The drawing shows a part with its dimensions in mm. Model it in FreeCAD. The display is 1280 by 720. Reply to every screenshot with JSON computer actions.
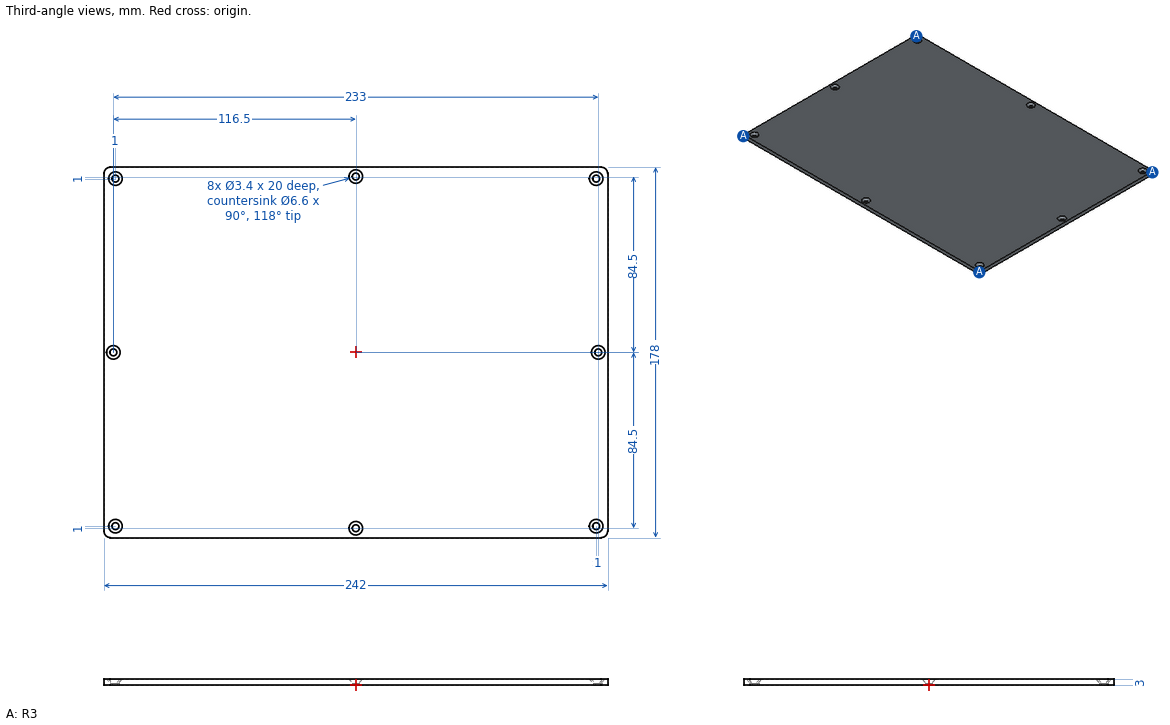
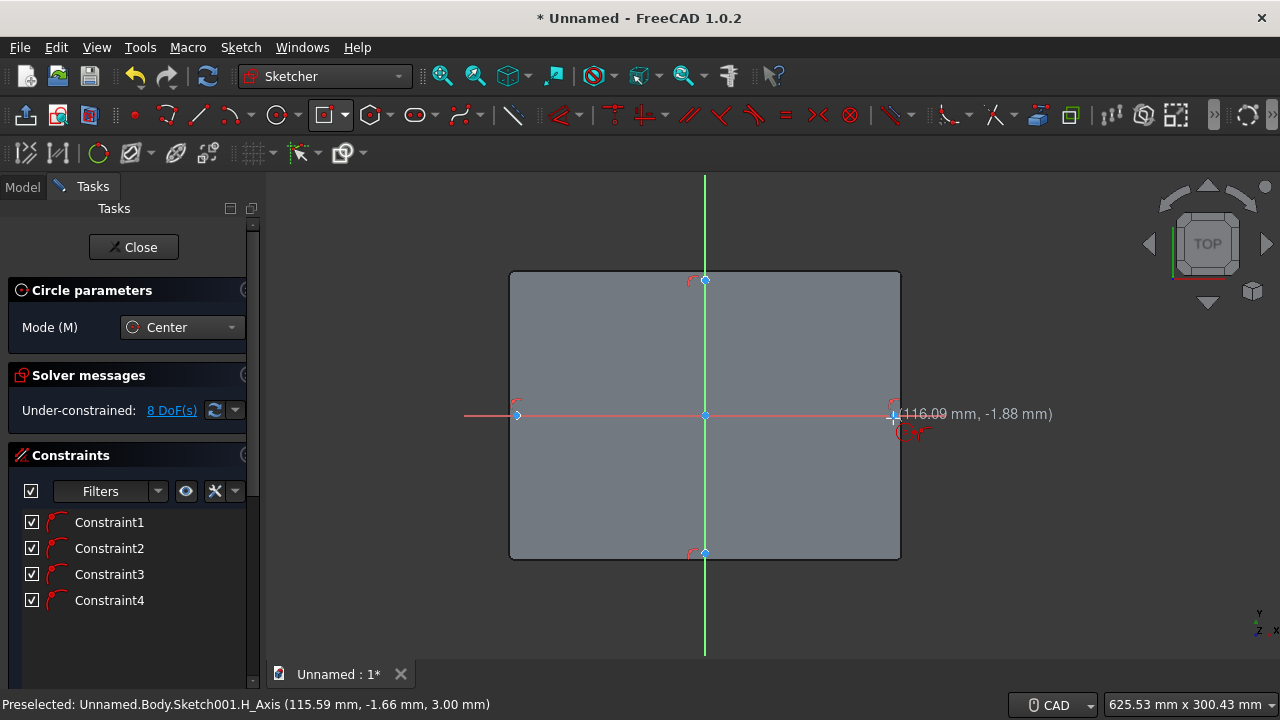
{"action": "scroll", "coordinate": [518, 280], "scroll_direction": "up", "scroll_amount": 11}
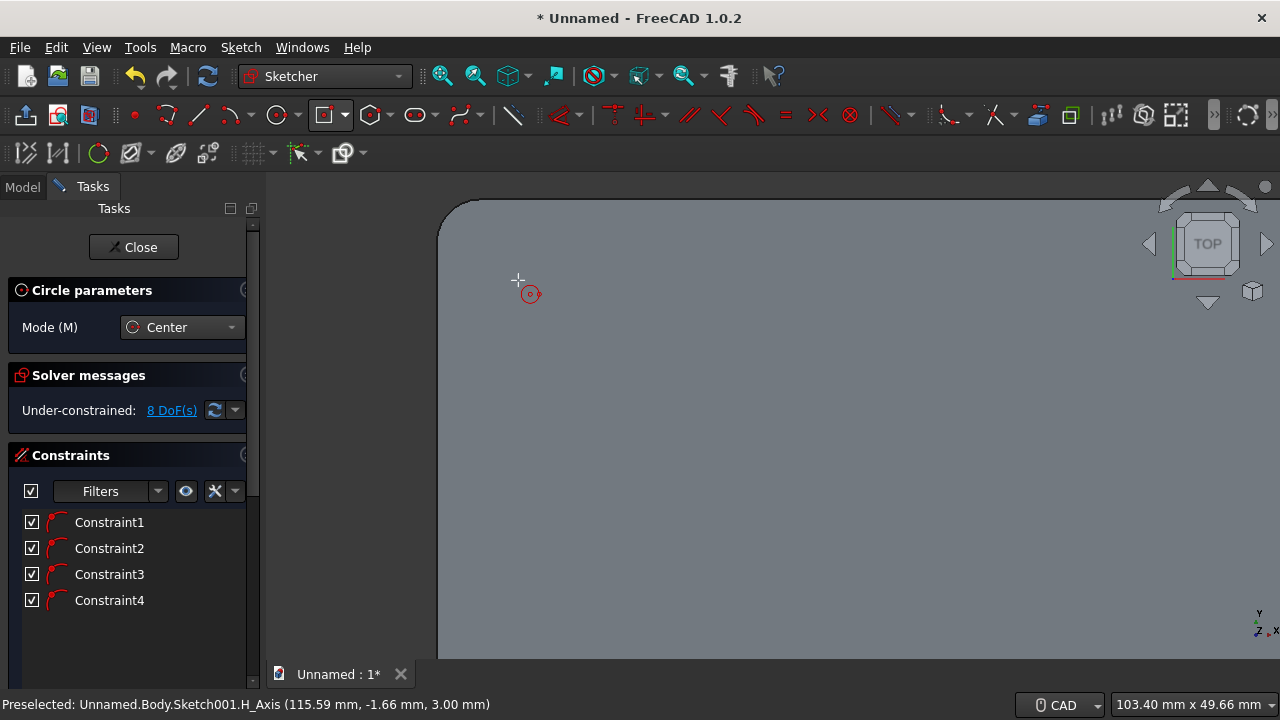
{"action": "scroll", "coordinate": [517, 280], "scroll_direction": "down", "scroll_amount": 11}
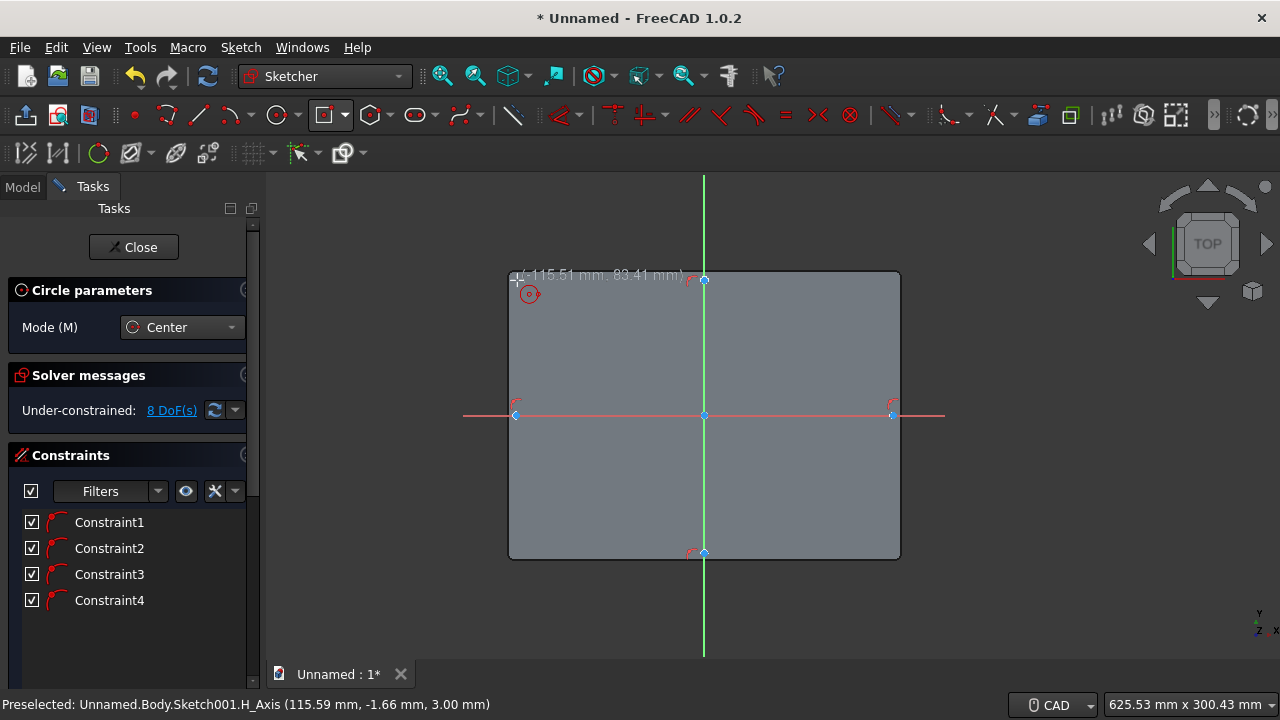
{"action": "left_click", "coordinate": [517, 280]}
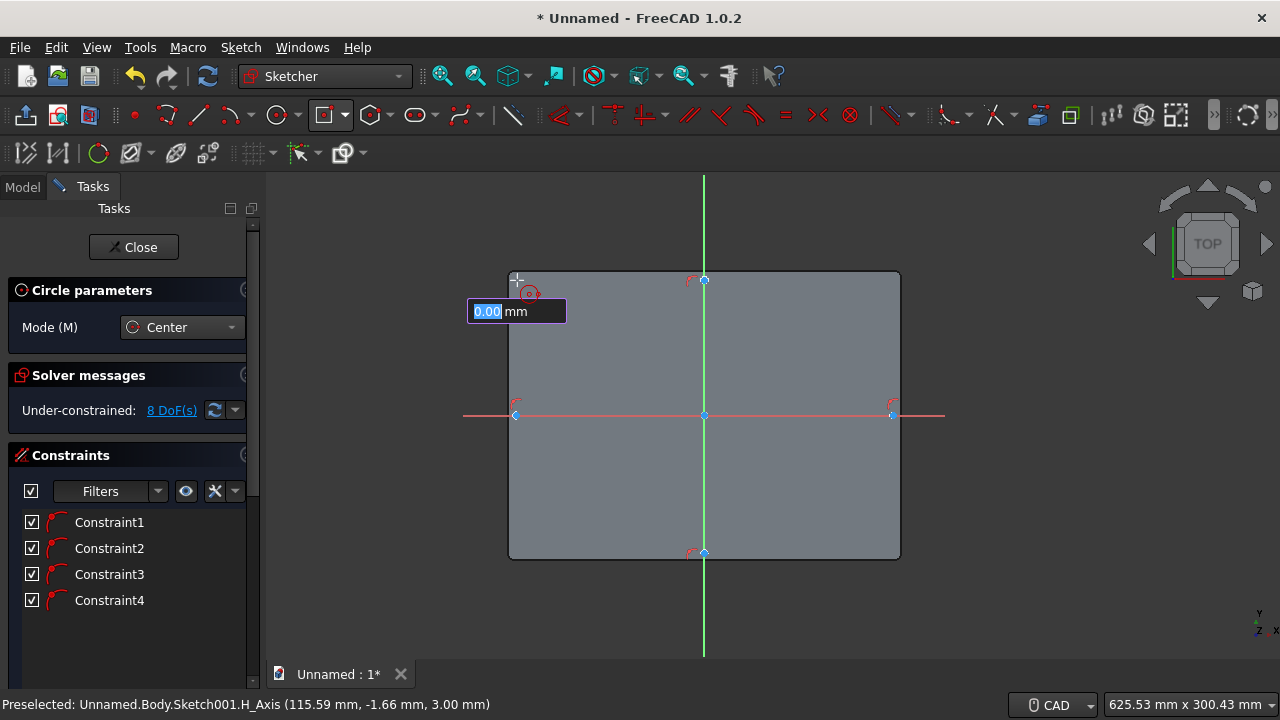
{"action": "scroll", "coordinate": [519, 278], "scroll_direction": "up", "scroll_amount": 9}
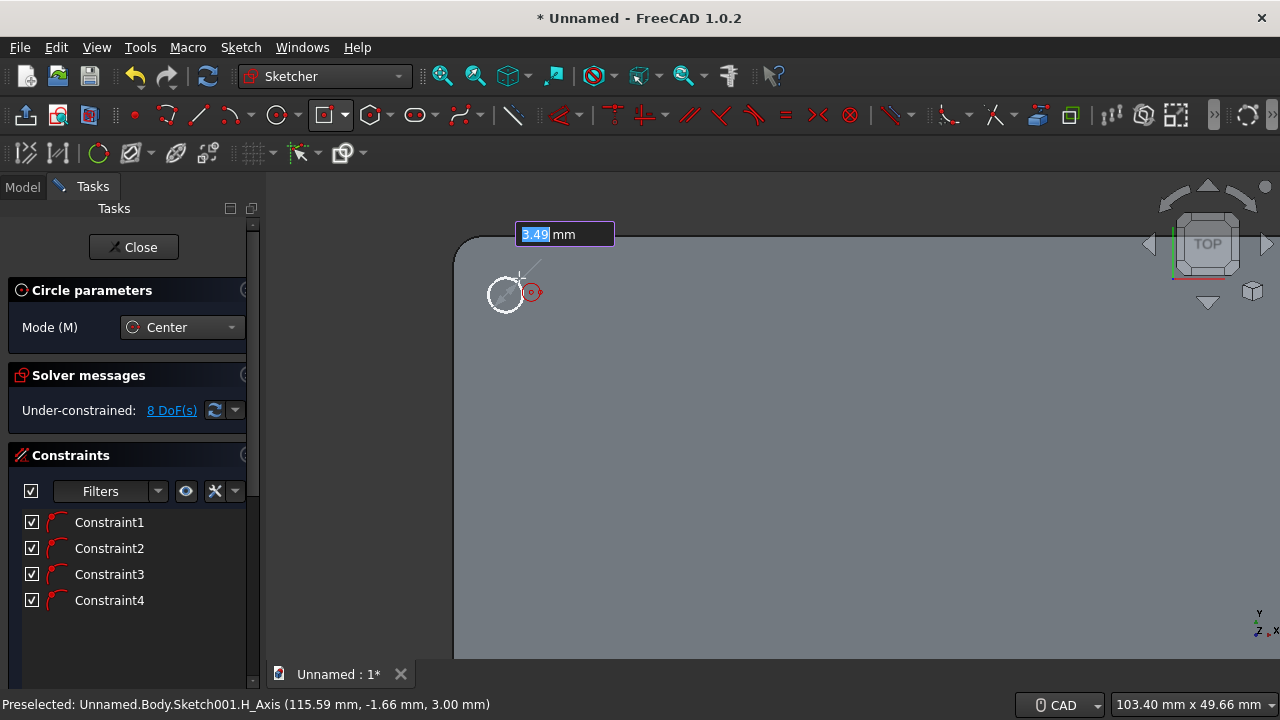
{"action": "left_click", "coordinate": [519, 278]}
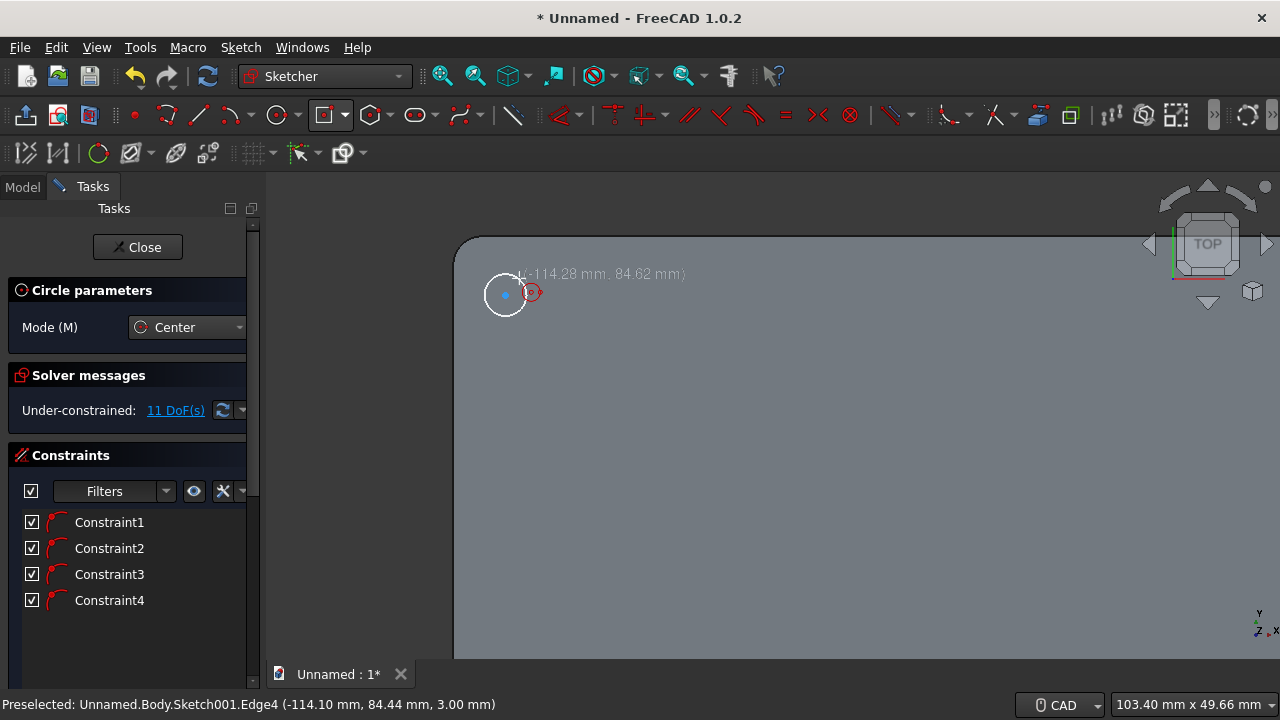
{"action": "scroll", "coordinate": [519, 278], "scroll_direction": "down", "scroll_amount": 9}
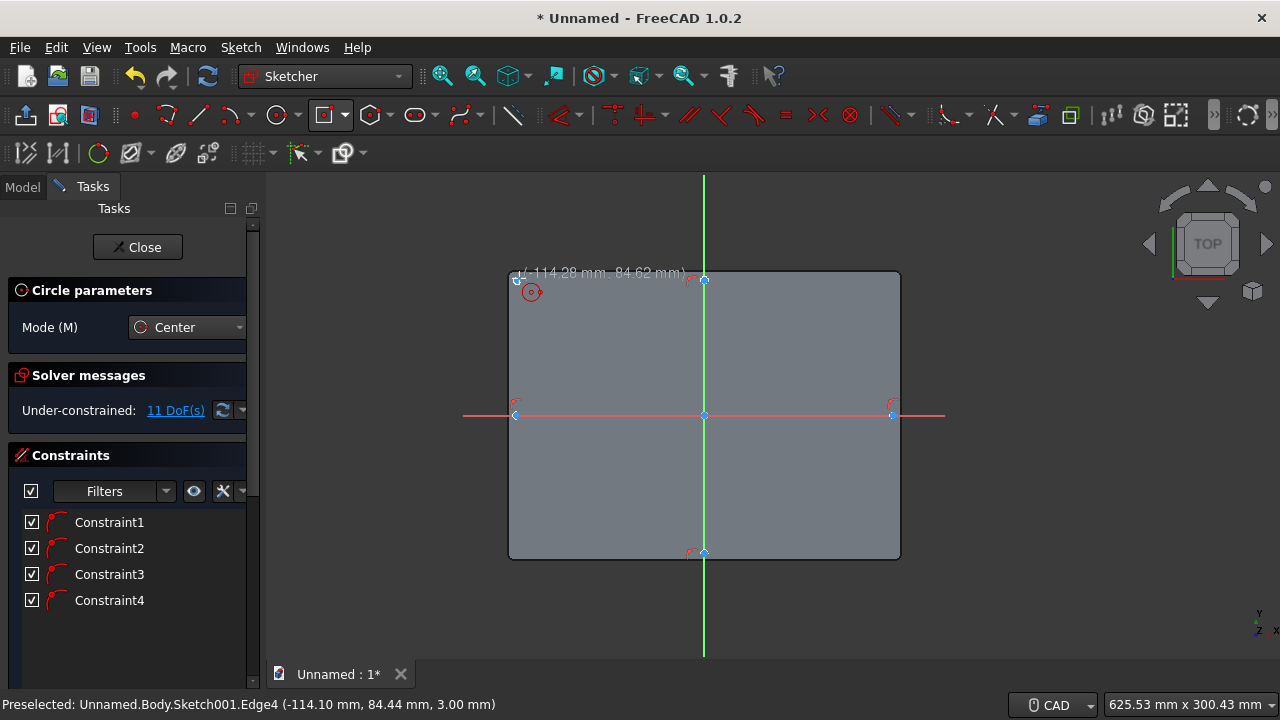
{"action": "scroll", "coordinate": [517, 551], "scroll_direction": "up", "scroll_amount": 11}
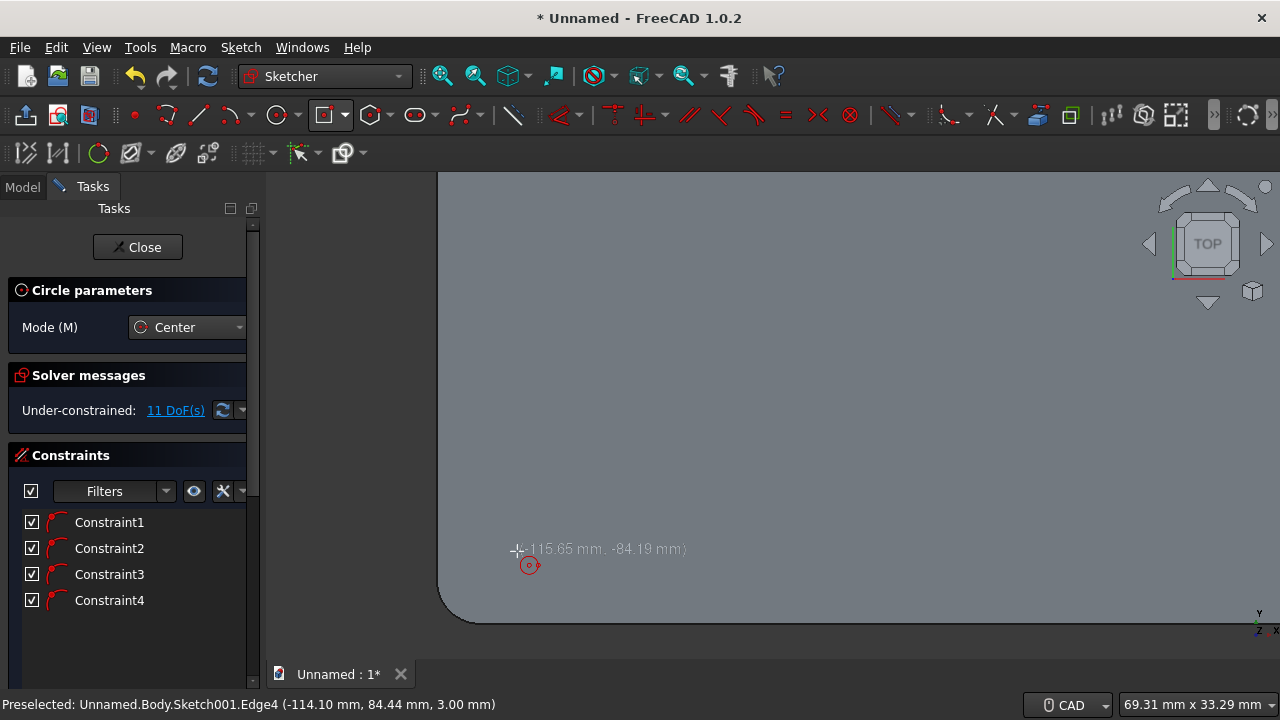
{"action": "scroll", "coordinate": [517, 552], "scroll_direction": "down", "scroll_amount": 11}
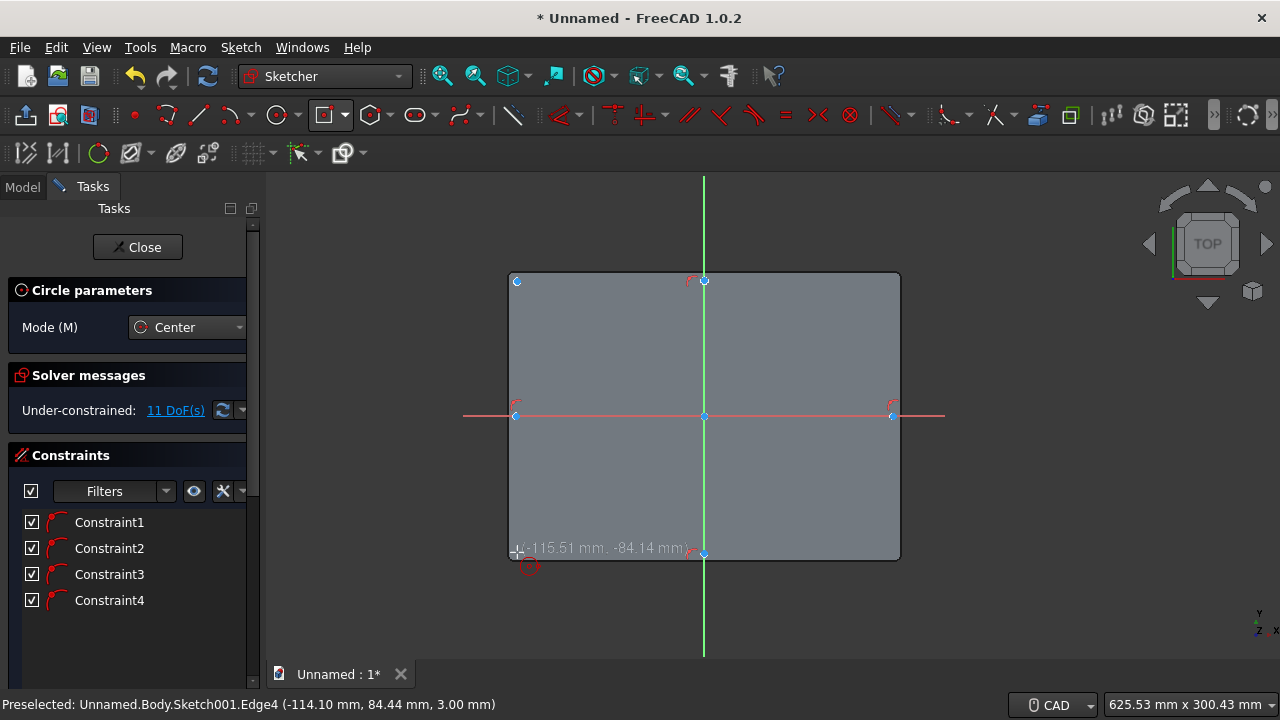
{"action": "left_click", "coordinate": [517, 552]}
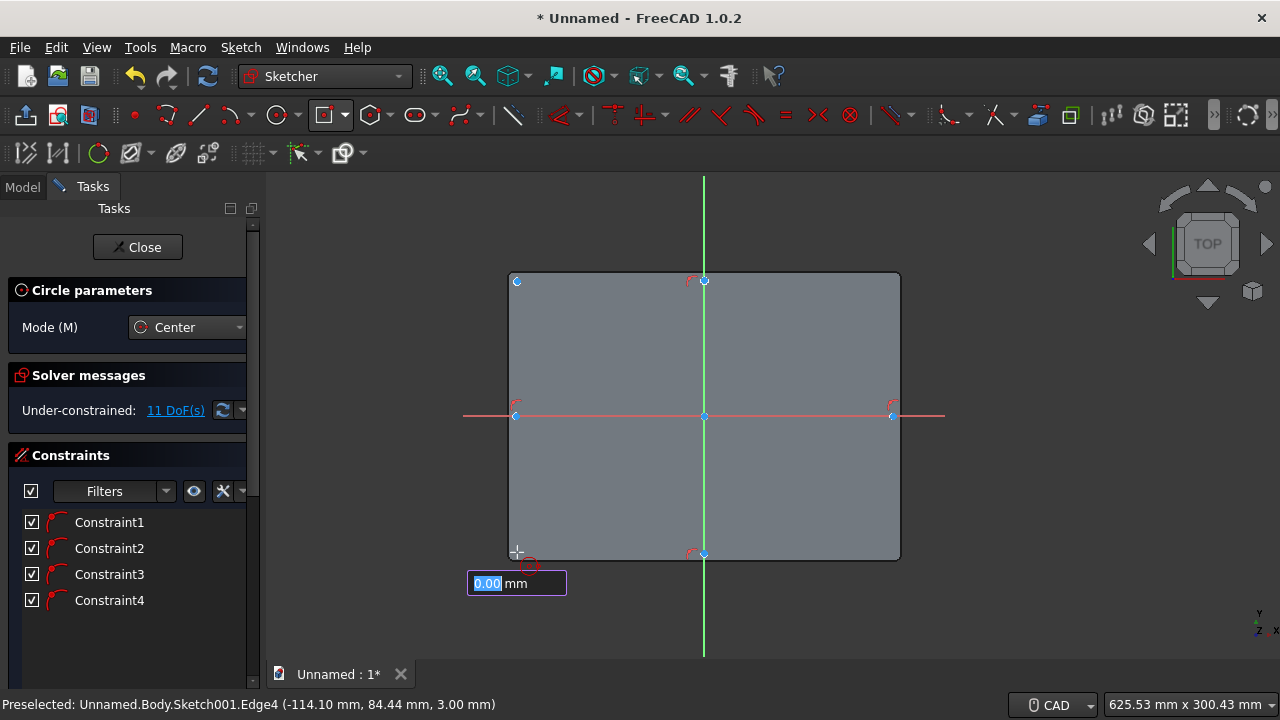
{"action": "scroll", "coordinate": [519, 550], "scroll_direction": "up", "scroll_amount": 9}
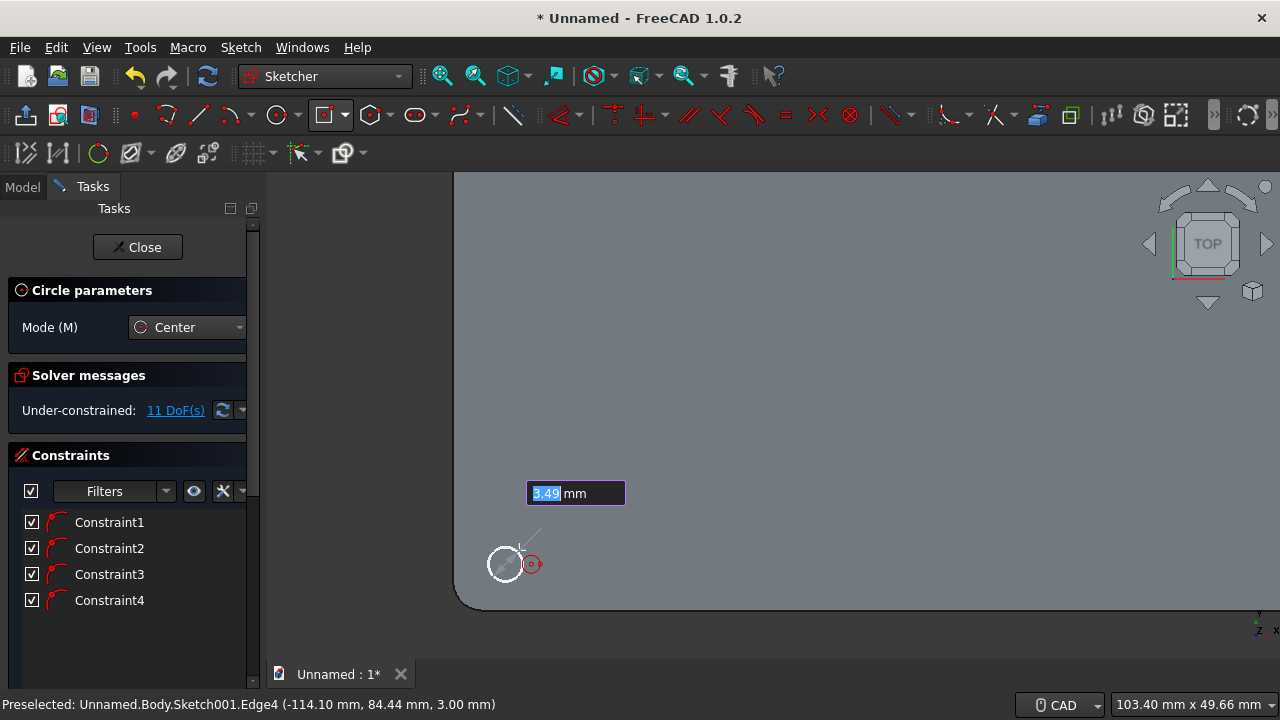
{"action": "left_click", "coordinate": [519, 545]}